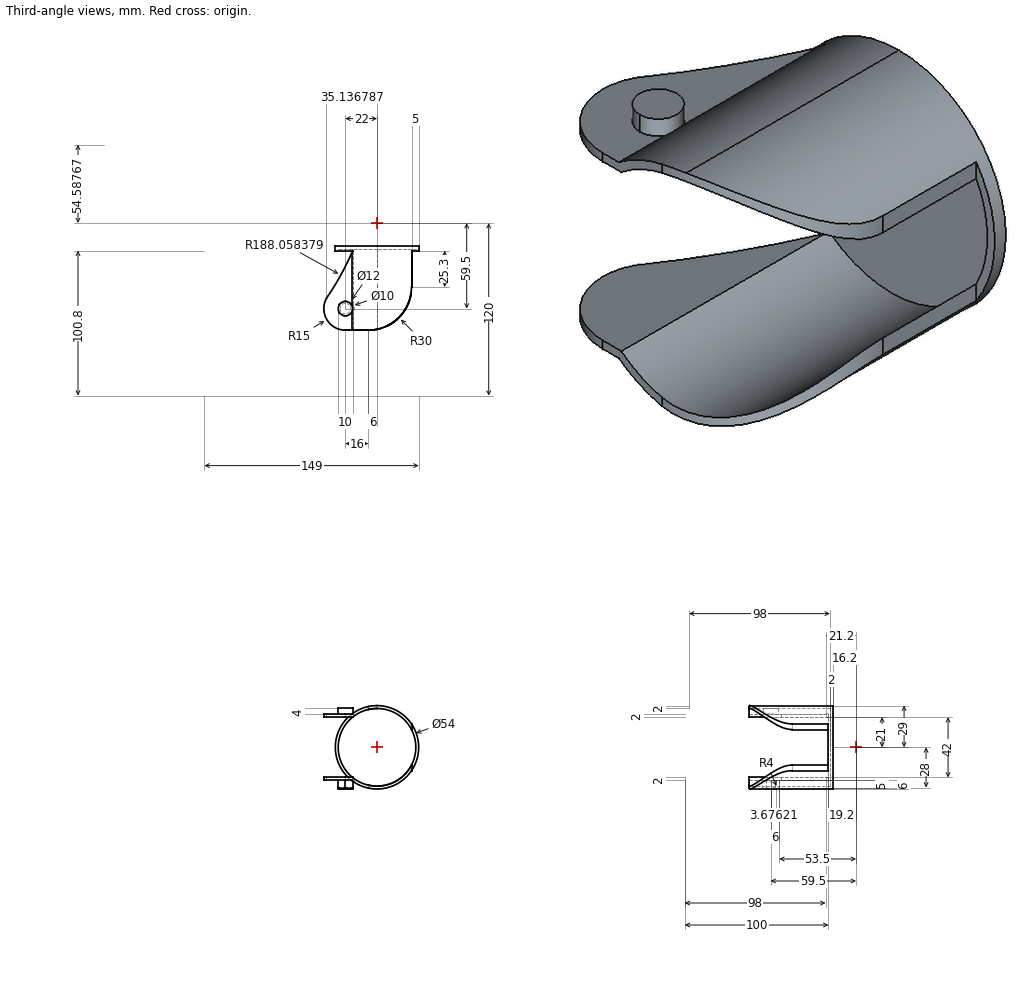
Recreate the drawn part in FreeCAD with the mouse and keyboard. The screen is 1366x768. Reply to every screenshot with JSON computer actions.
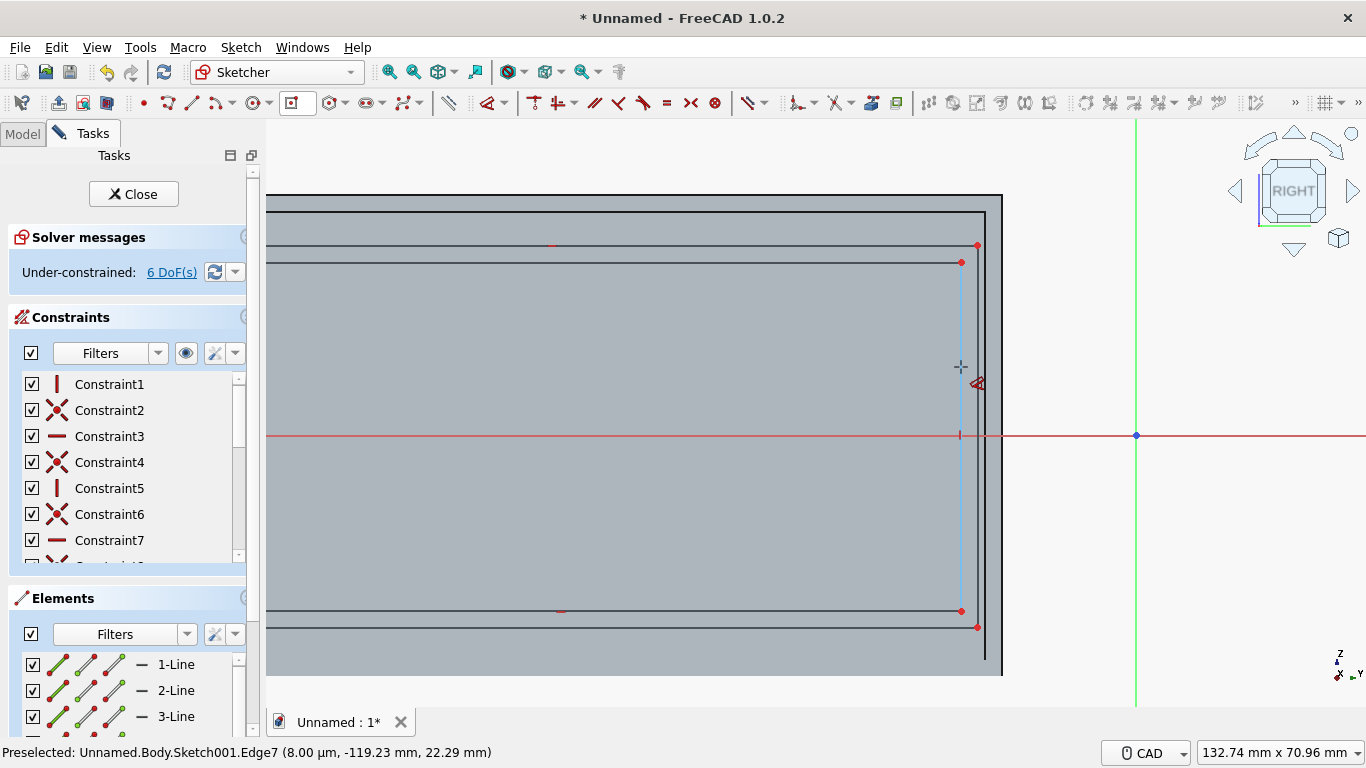
{"action": "left_click", "coordinate": [961, 367]}
{"action": "left_click", "coordinate": [995, 357]}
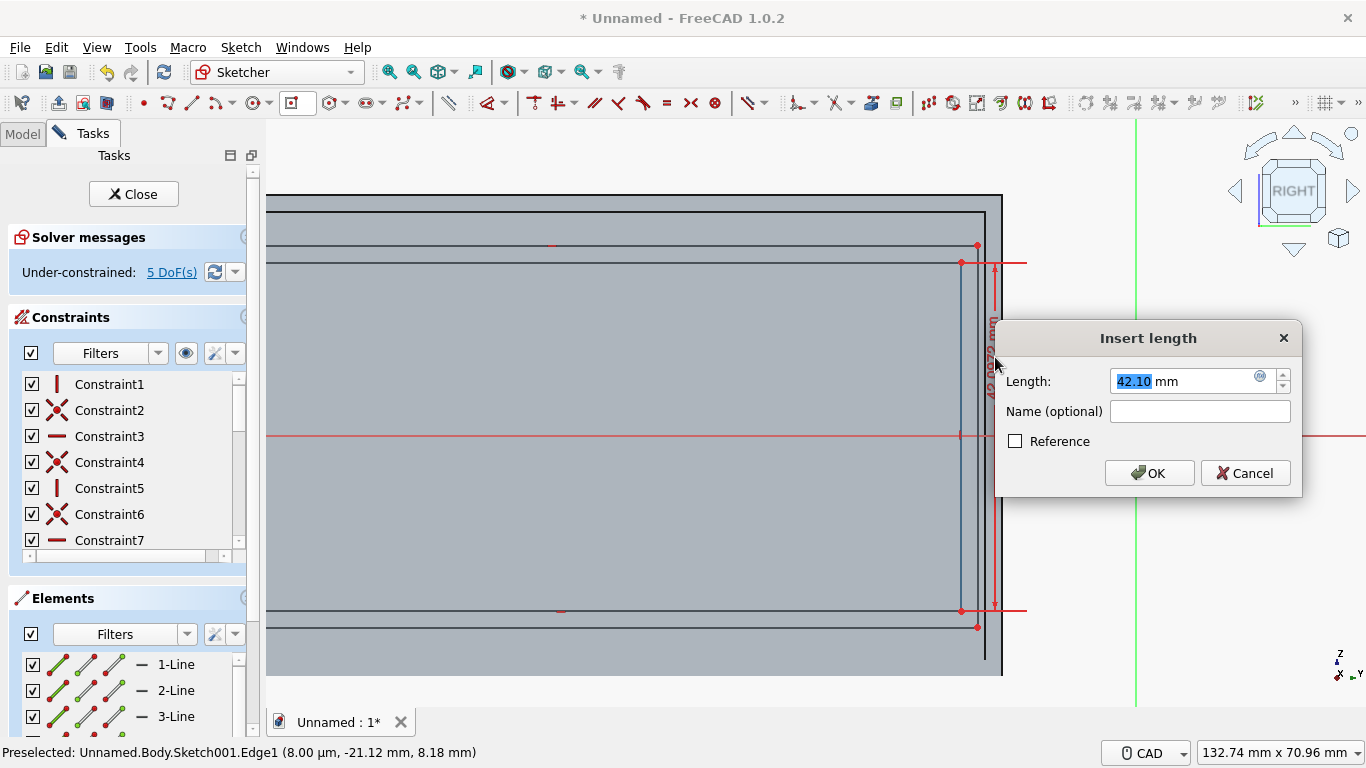
{"action": "type", "text": "42"}
{"action": "key", "text": "Return"}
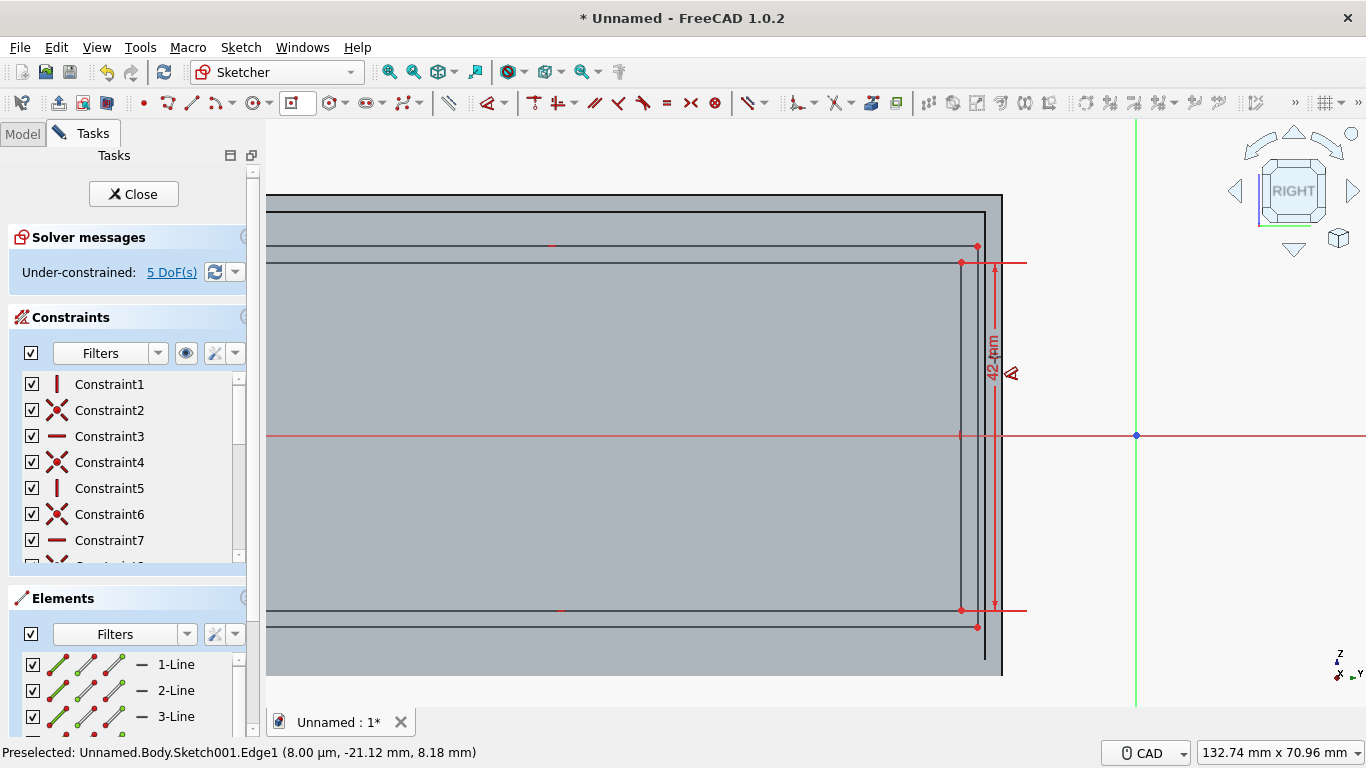
{"action": "left_click", "coordinate": [717, 611]}
{"action": "left_click", "coordinate": [628, 645]}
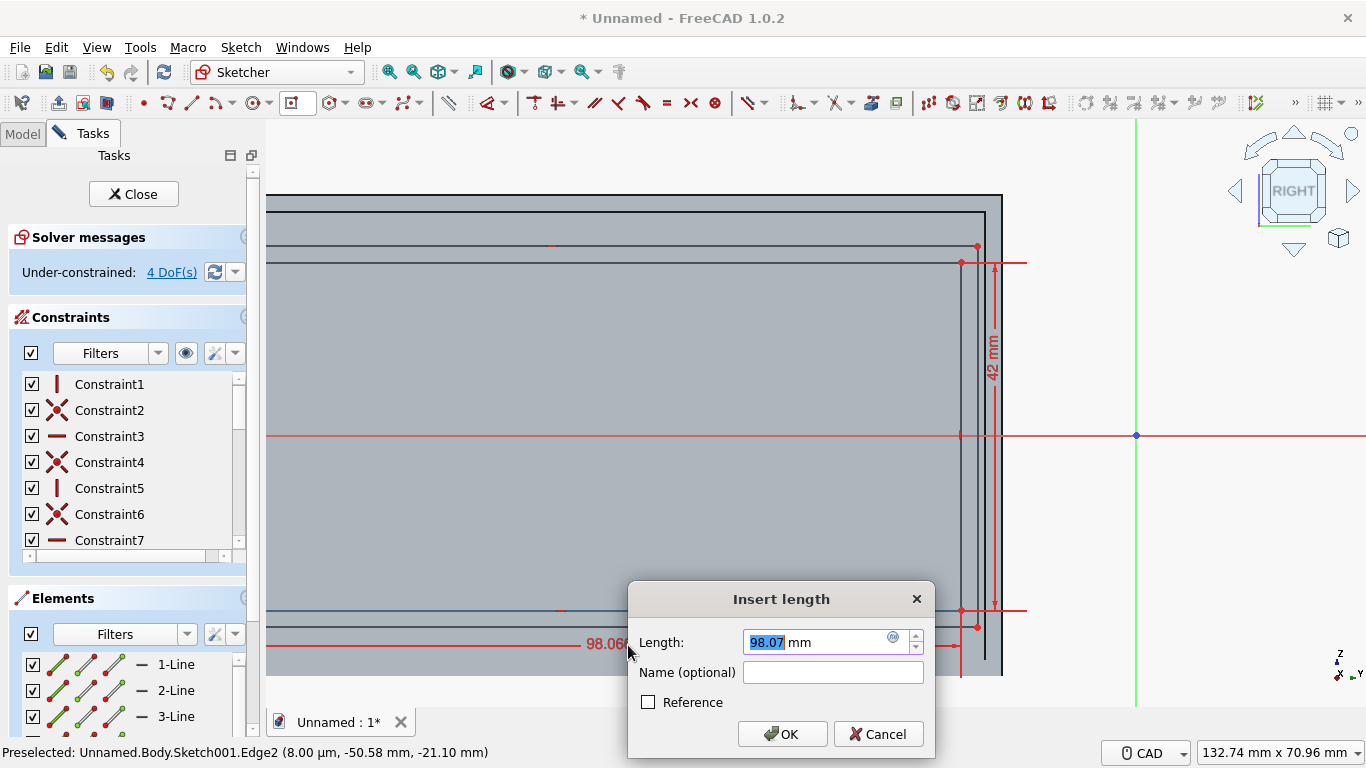
{"action": "type", "text": "98"}
{"action": "key", "text": "Return"}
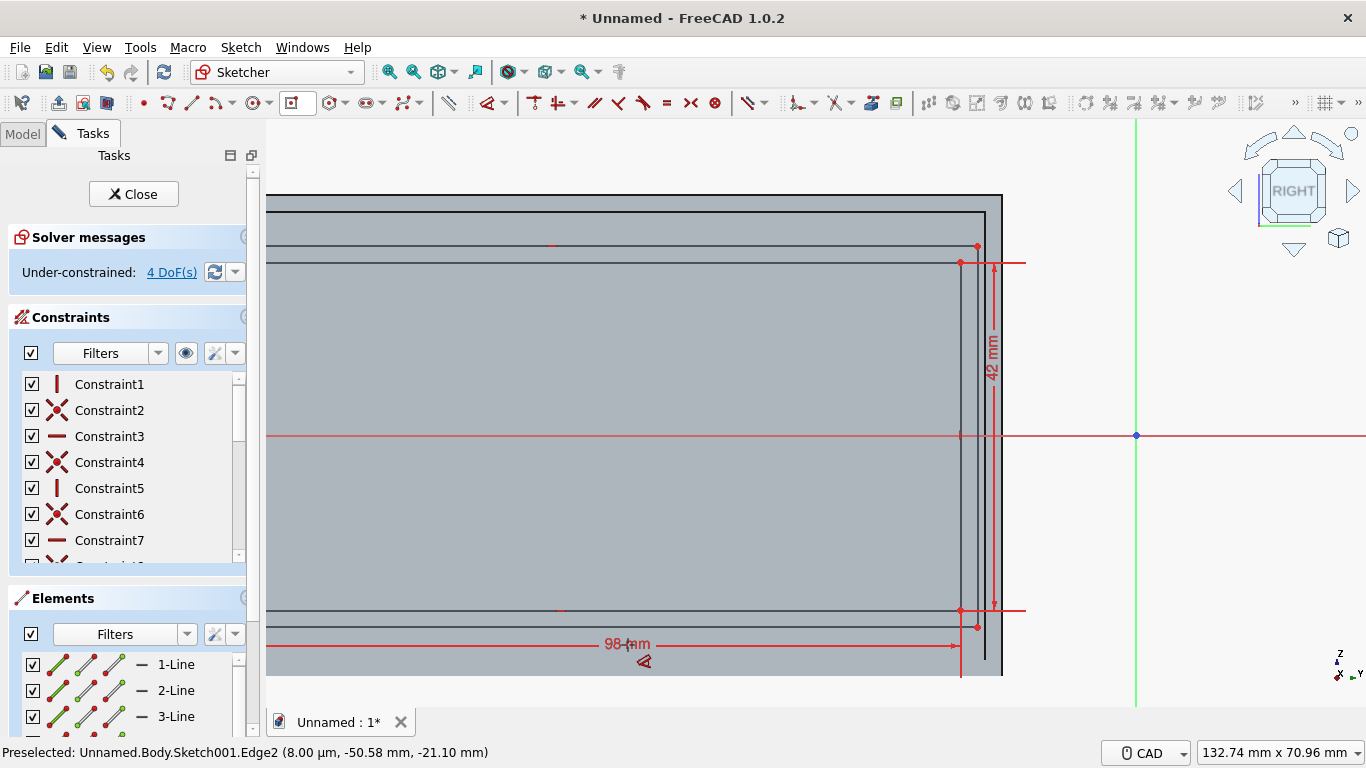
{"action": "left_click", "coordinate": [392, 263]}
{"action": "left_click", "coordinate": [627, 229]}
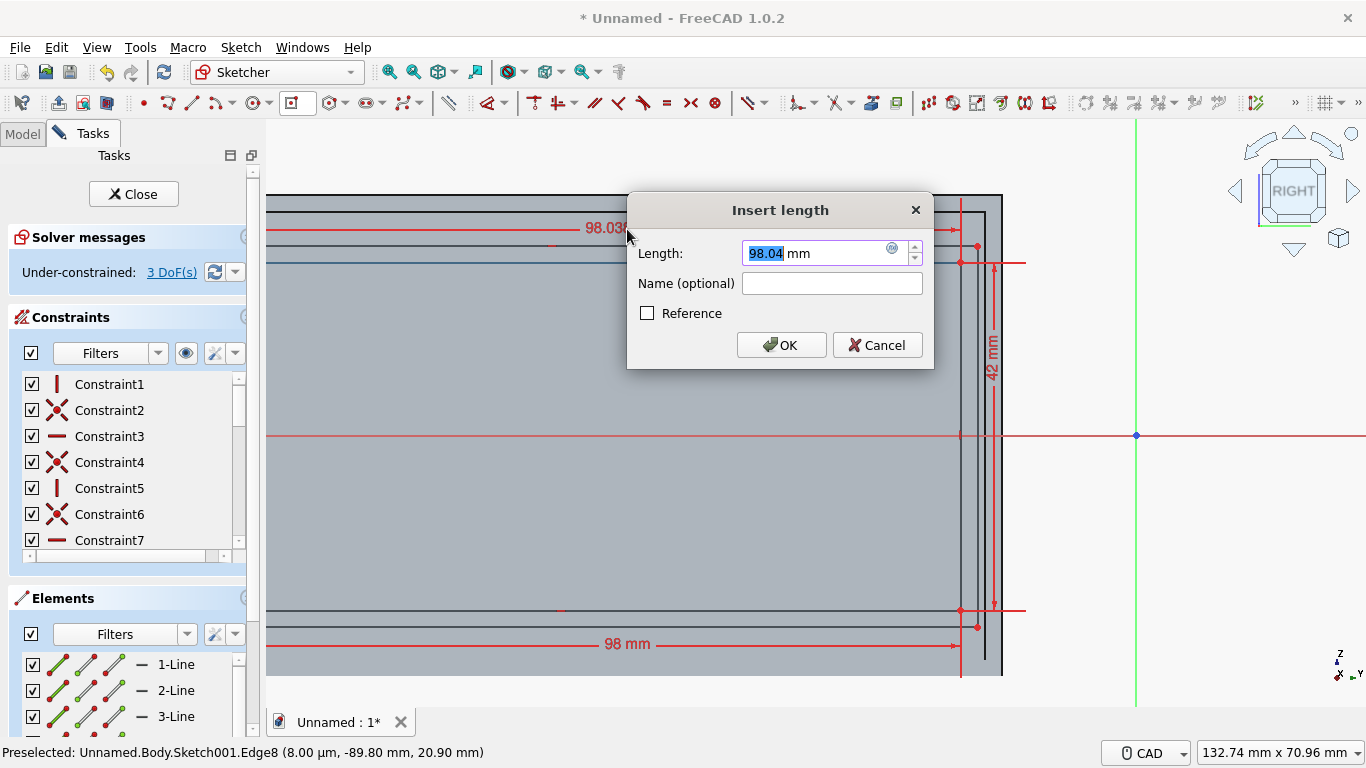
{"action": "type", "text": "98"}
{"action": "key", "text": "Return"}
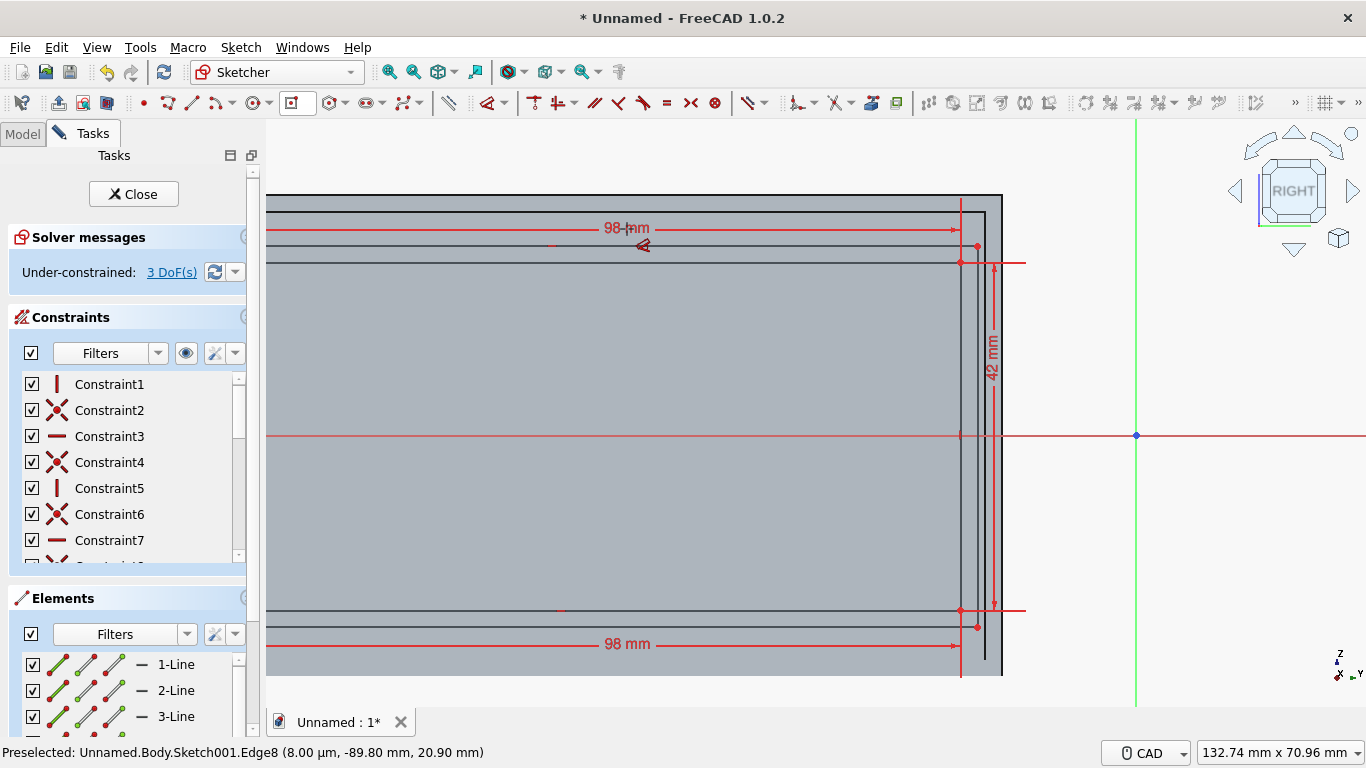
{"action": "left_click", "coordinate": [397, 627]}
{"action": "left_click", "coordinate": [479, 661]}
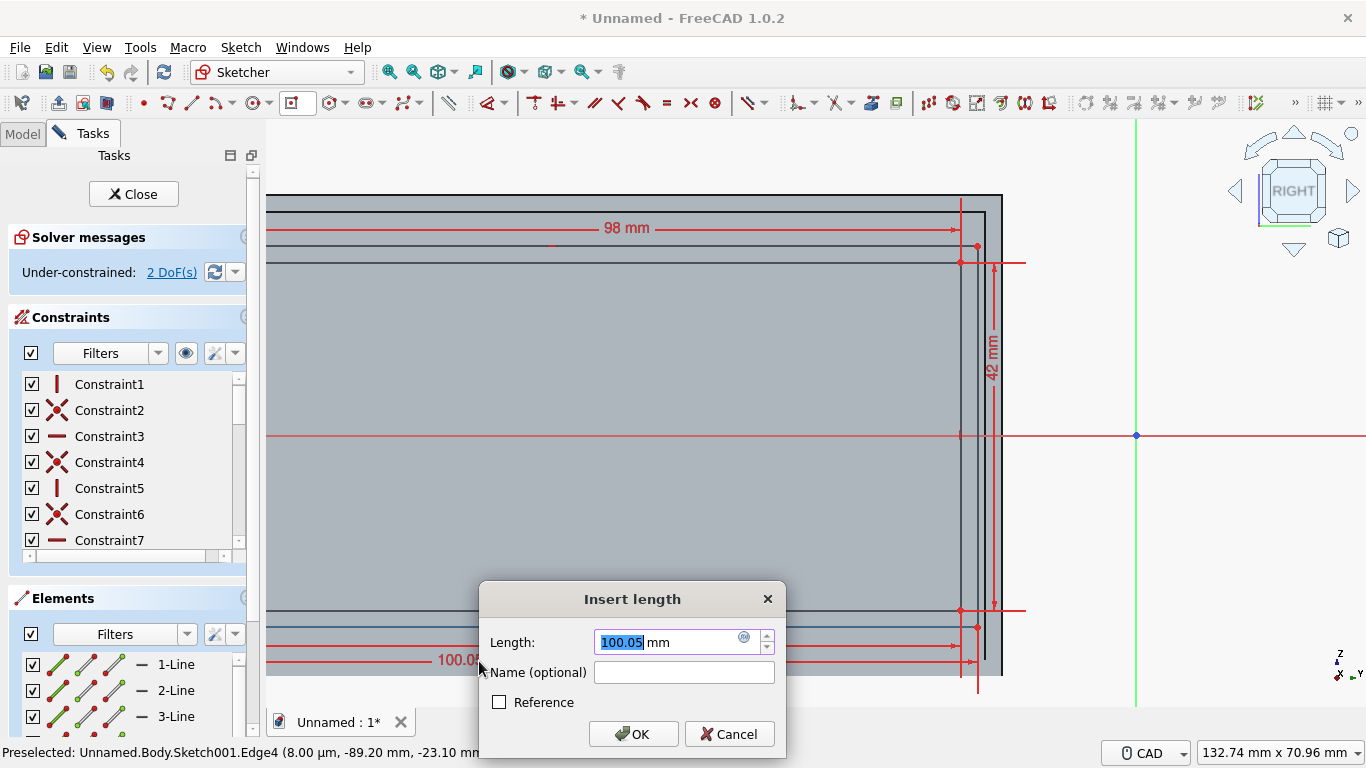
{"action": "type", "text": "100"}
{"action": "key", "text": "Return"}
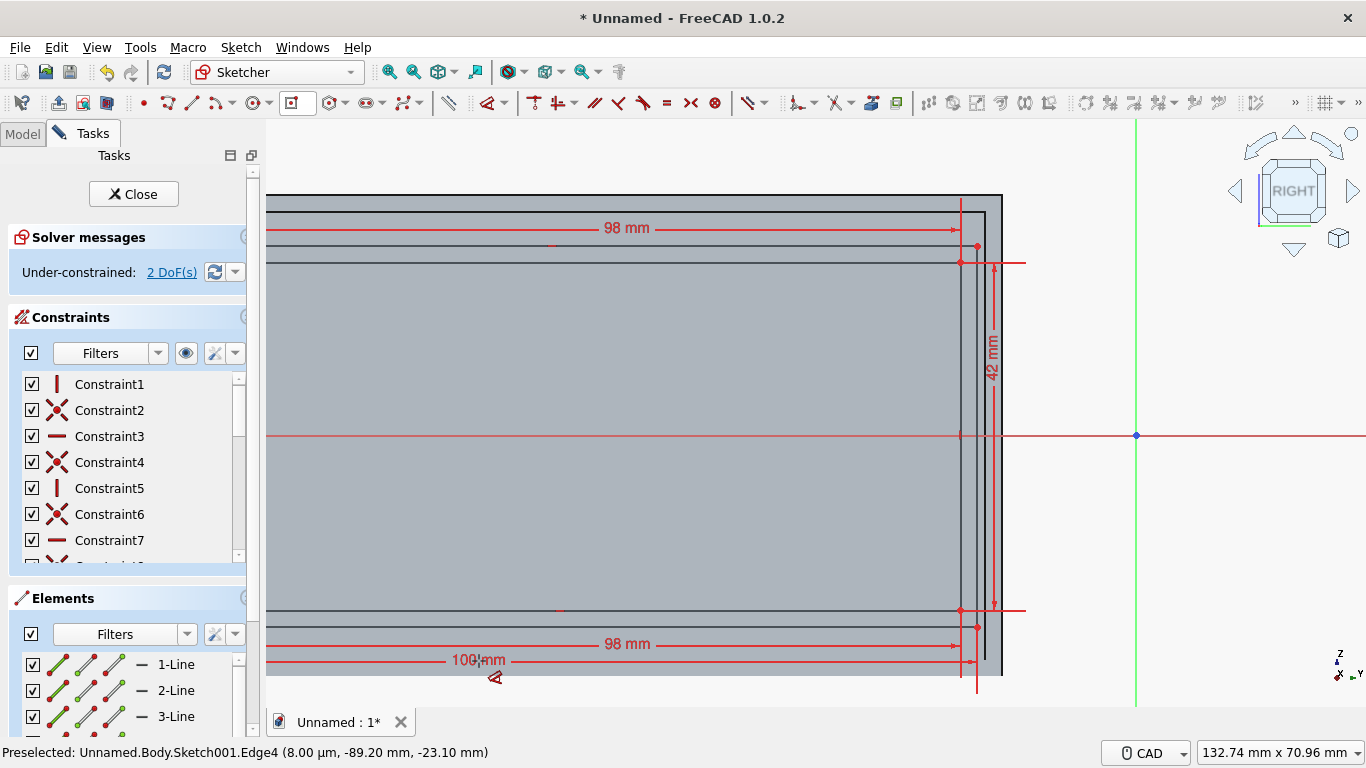
{"action": "left_click", "coordinate": [961, 263]}
{"action": "left_click", "coordinate": [1170, 349]}